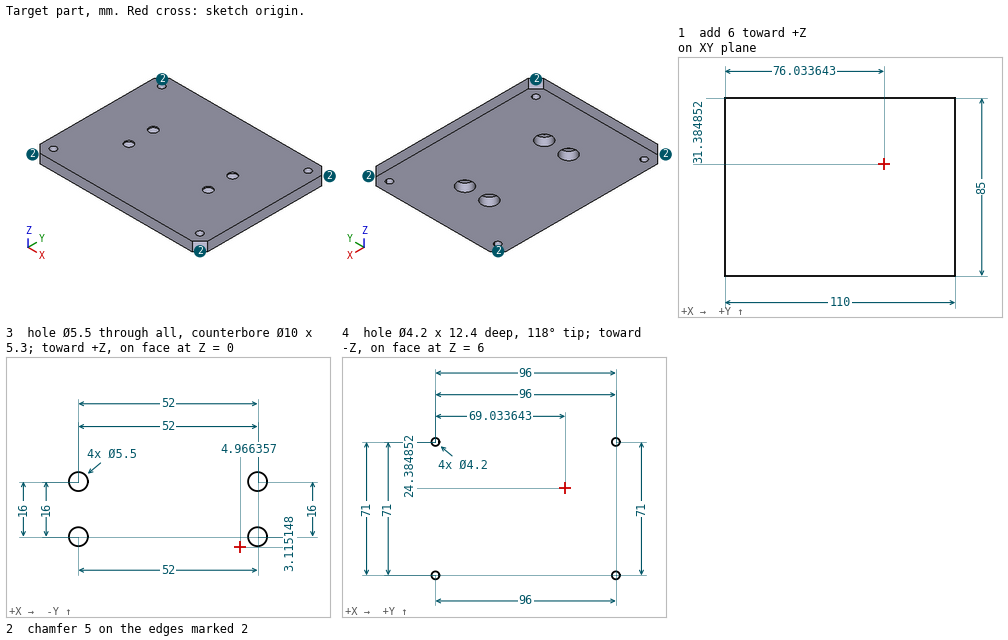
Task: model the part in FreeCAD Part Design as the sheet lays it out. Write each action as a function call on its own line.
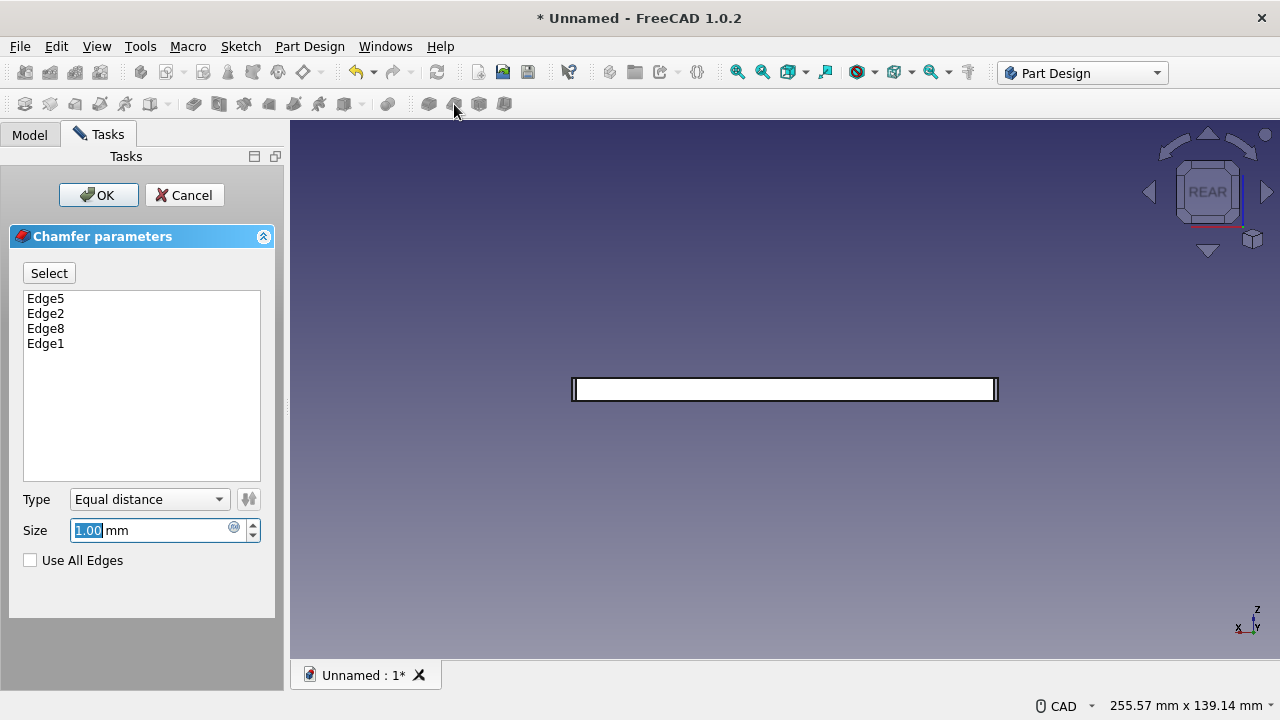
text(5)
key(Tab)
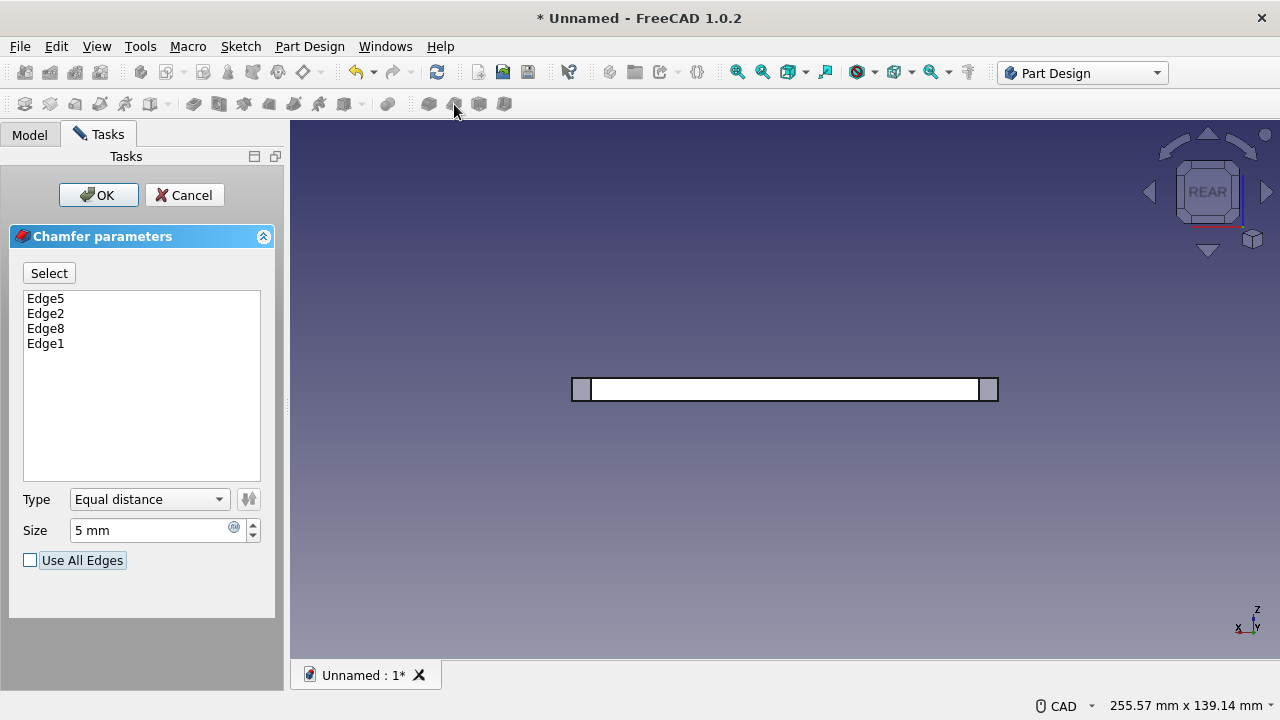
click(99, 195)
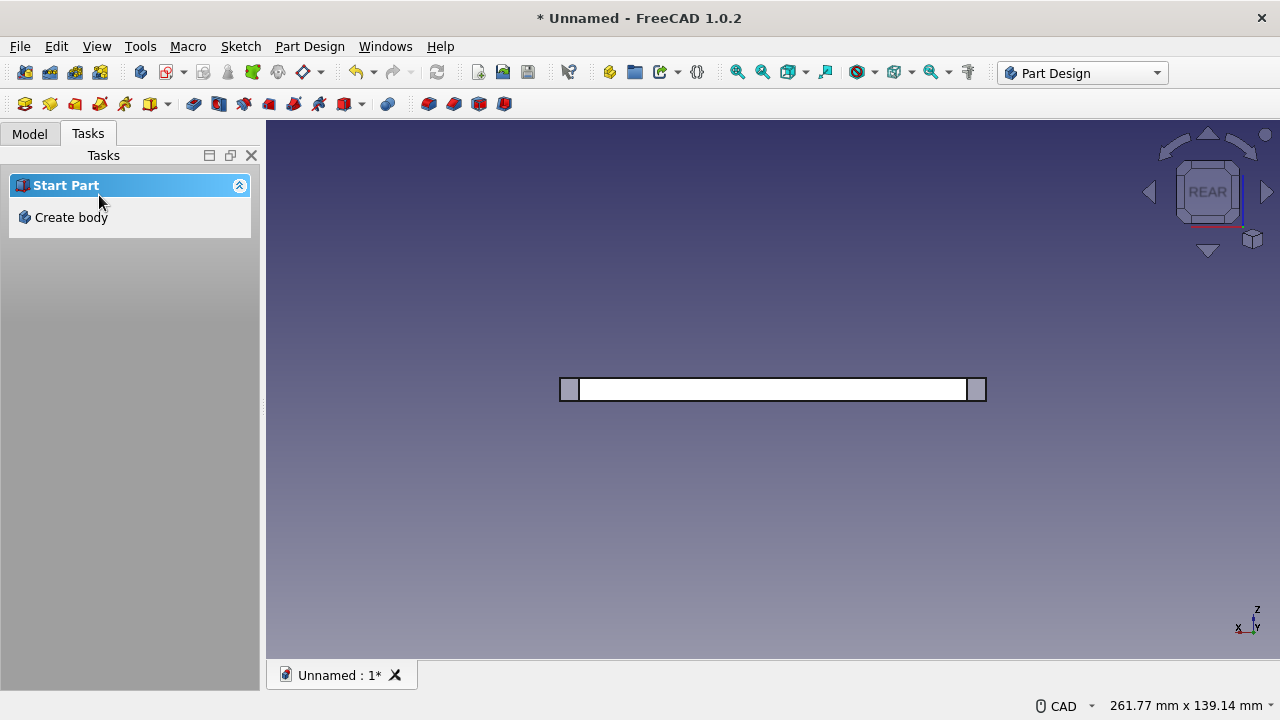
click(738, 72)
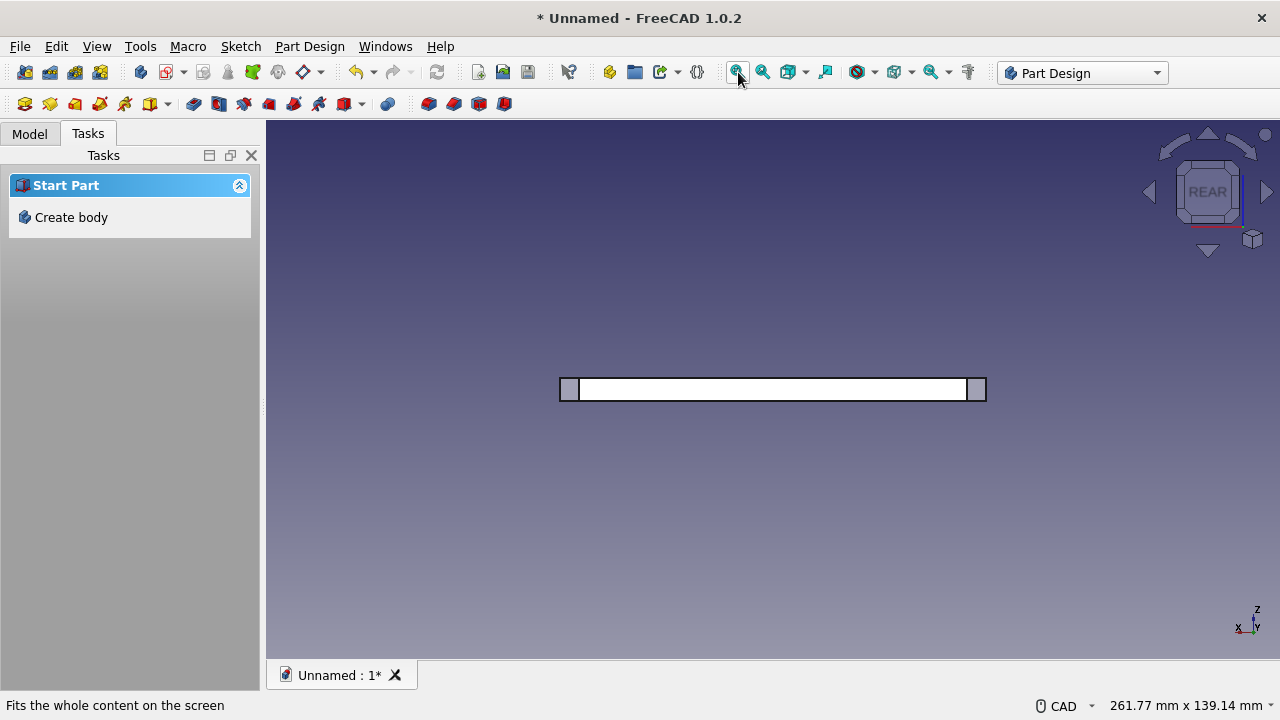
key(5)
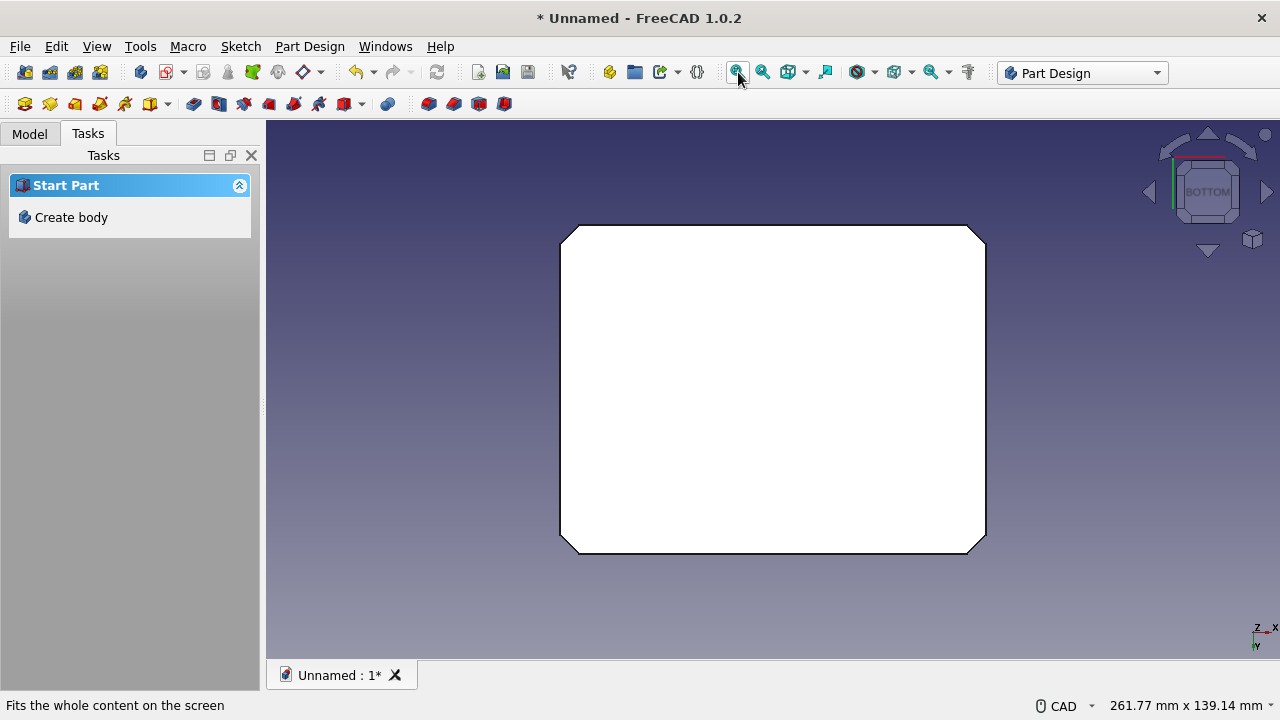
click(773, 388)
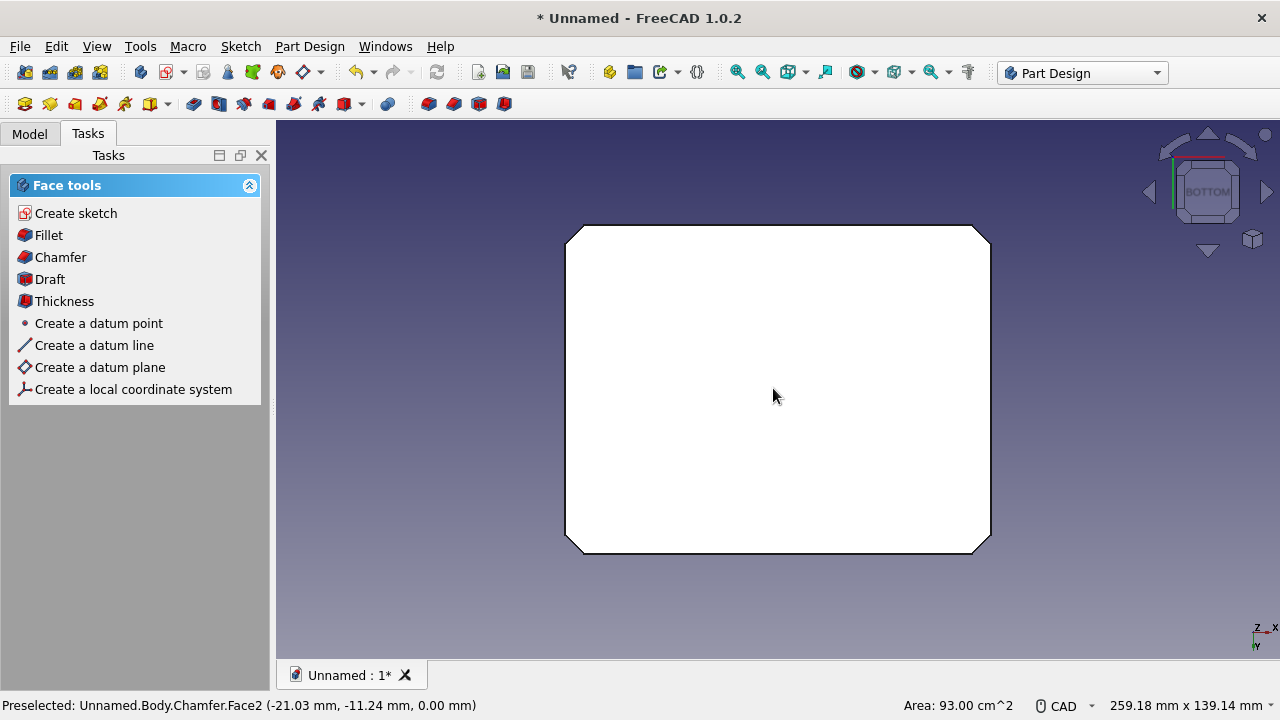
click(166, 72)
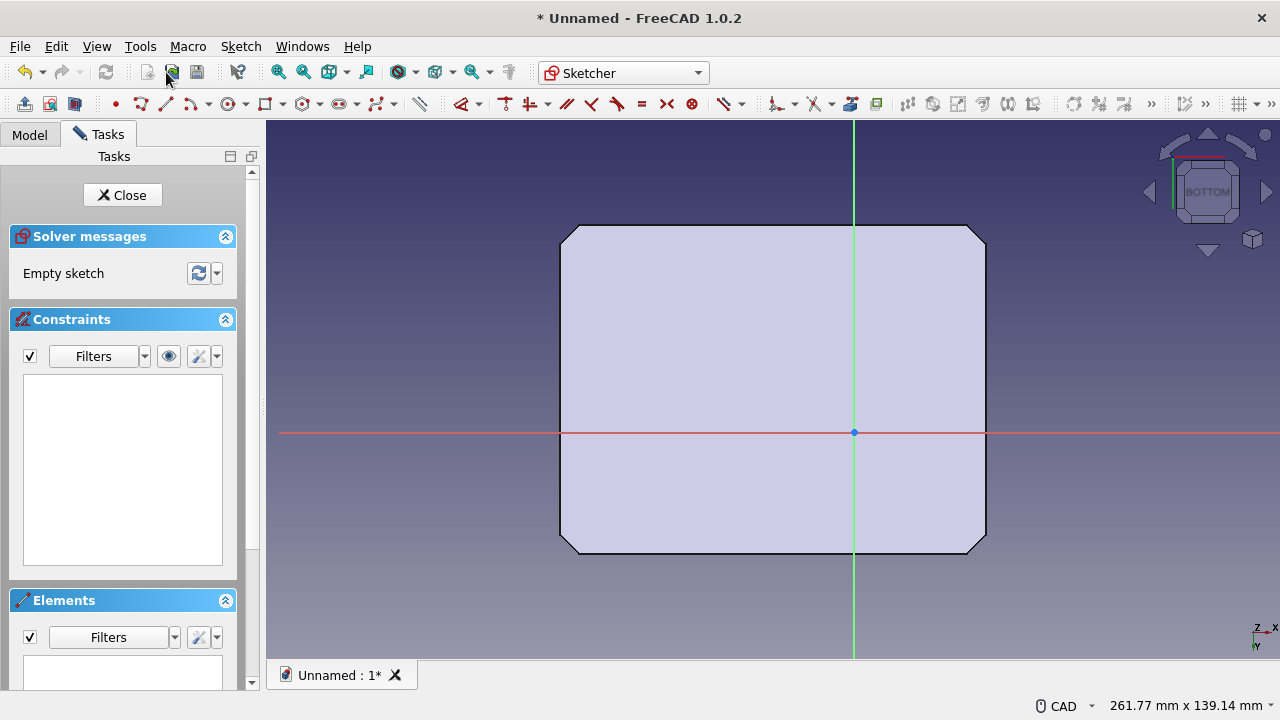
scroll(813, 391, up, 5)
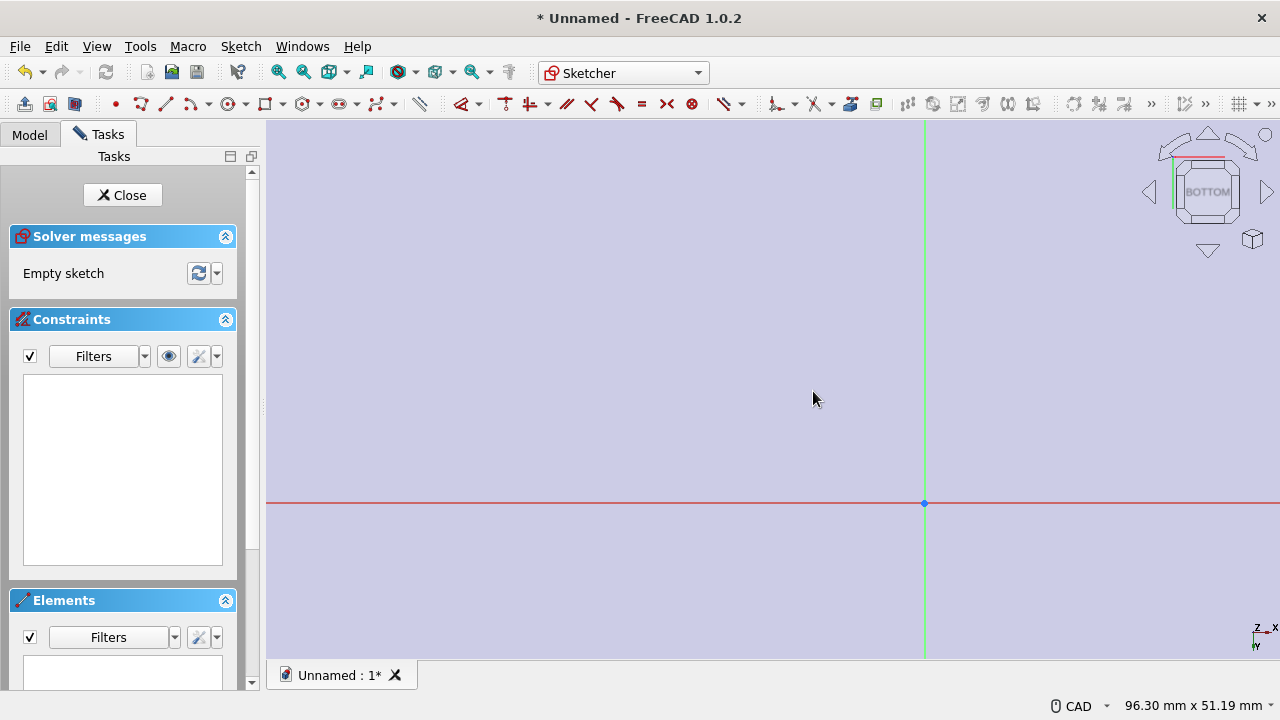
click(228, 104)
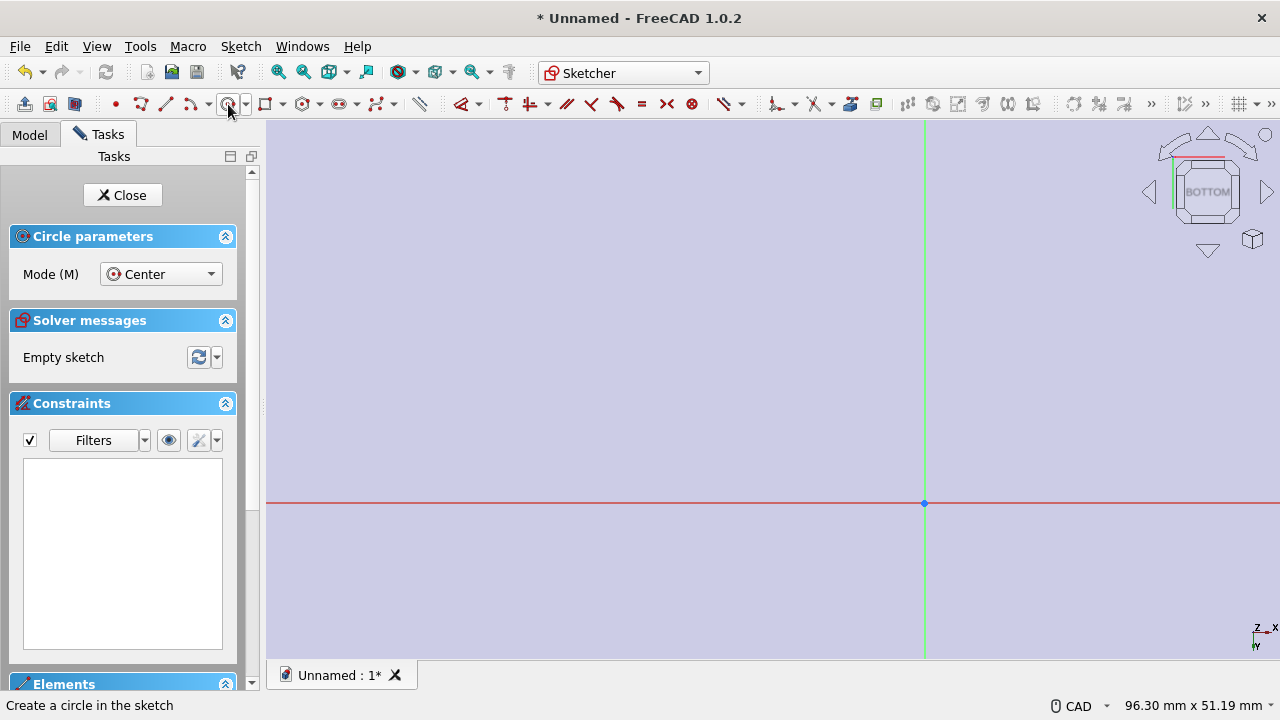
click(430, 302)
move(450, 281)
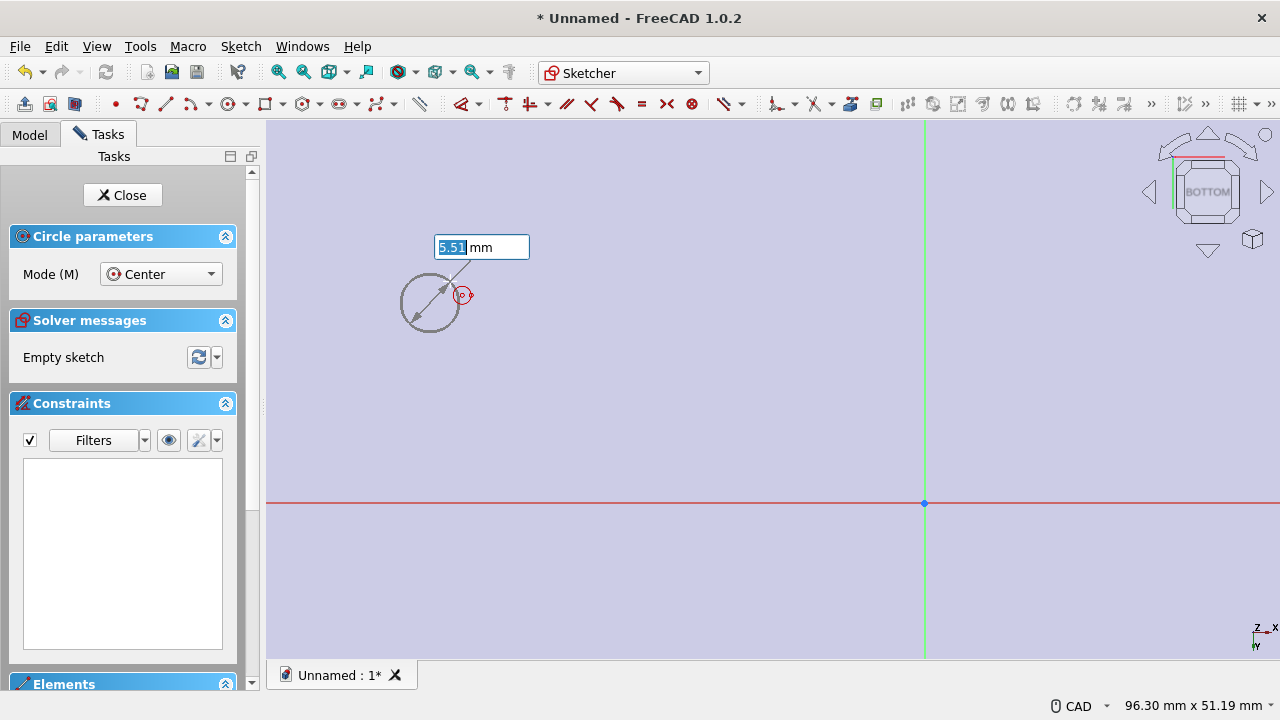
text(5.5)
key(Return)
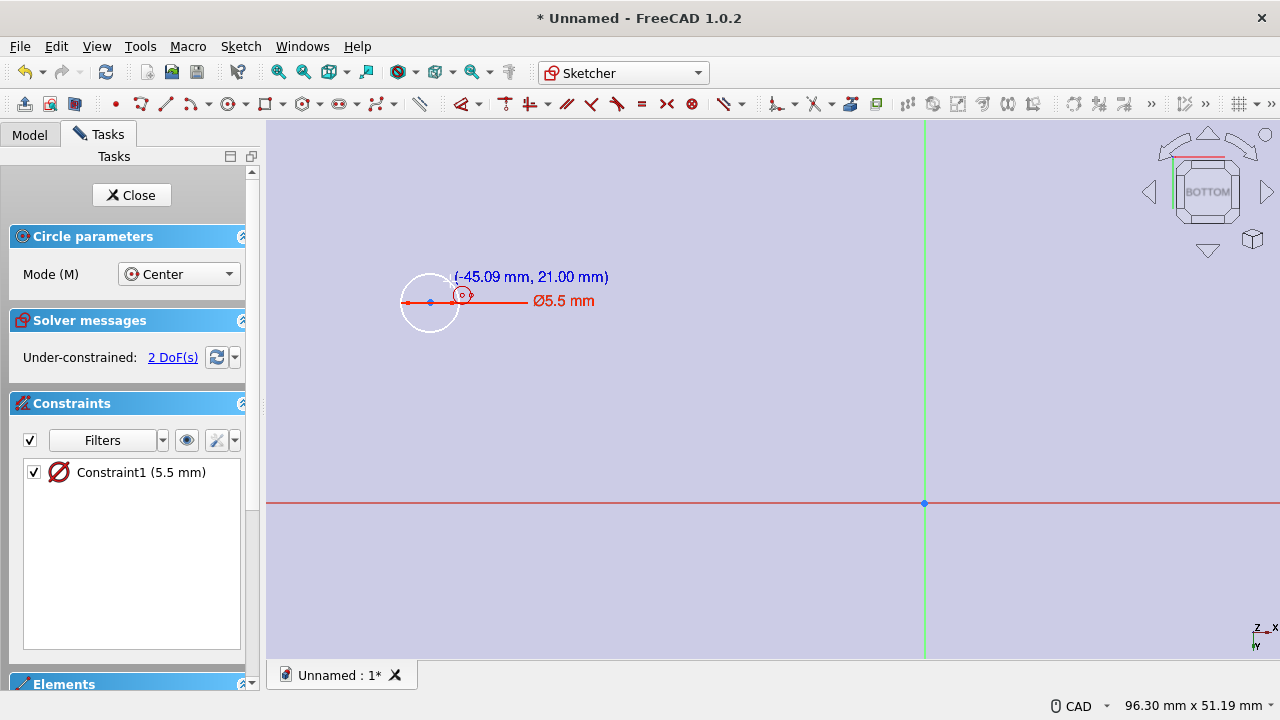
click(977, 302)
move(998, 281)